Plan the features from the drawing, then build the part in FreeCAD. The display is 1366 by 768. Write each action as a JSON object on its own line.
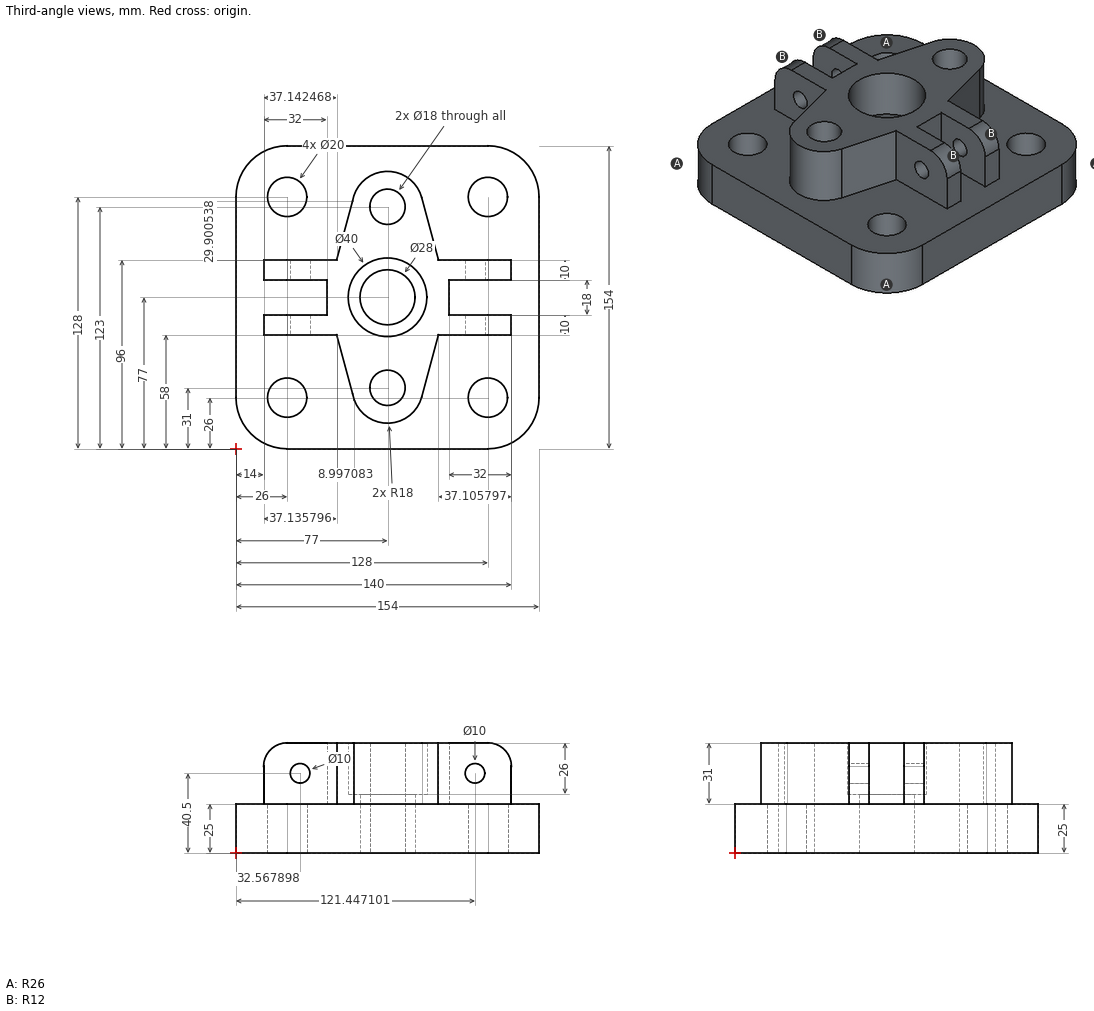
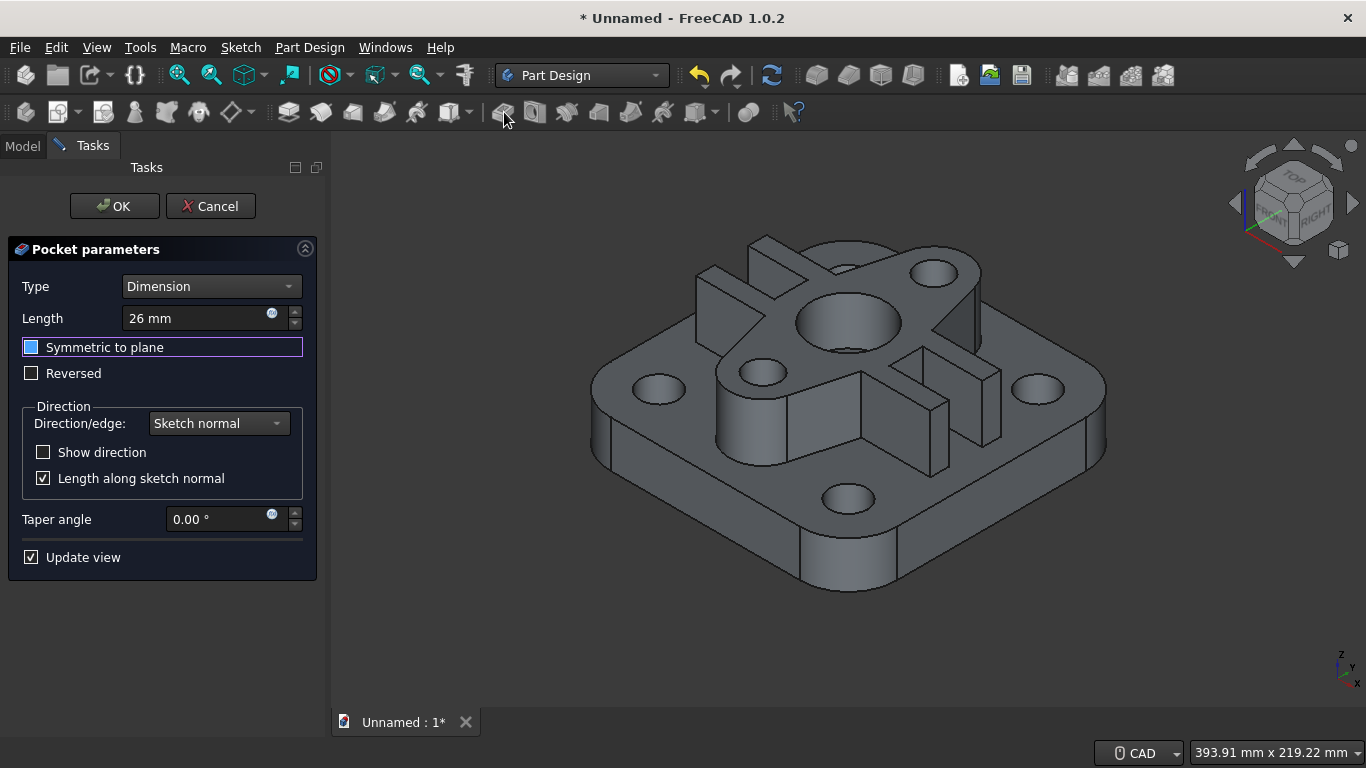
{"action": "left_click", "coordinate": [115, 206]}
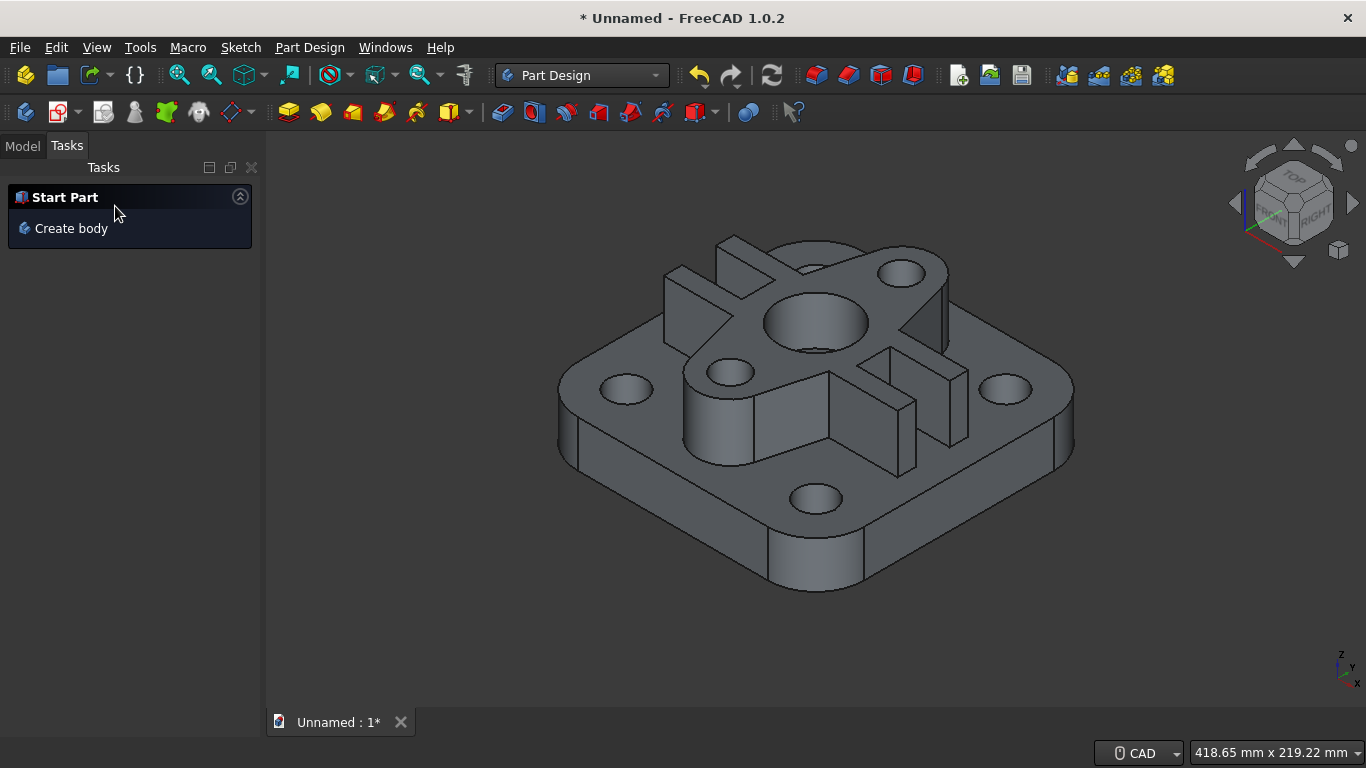
{"action": "left_click", "coordinate": [698, 328]}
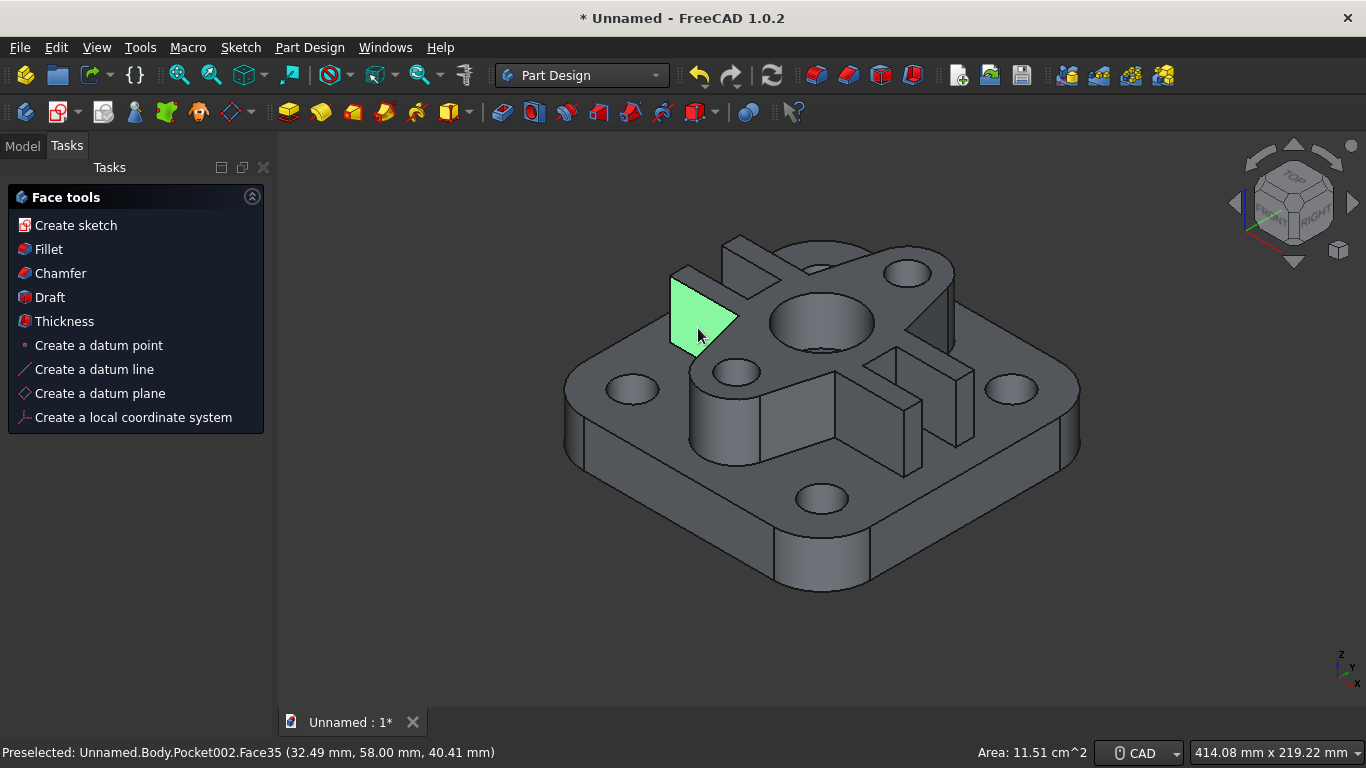
{"action": "left_click", "coordinate": [58, 112]}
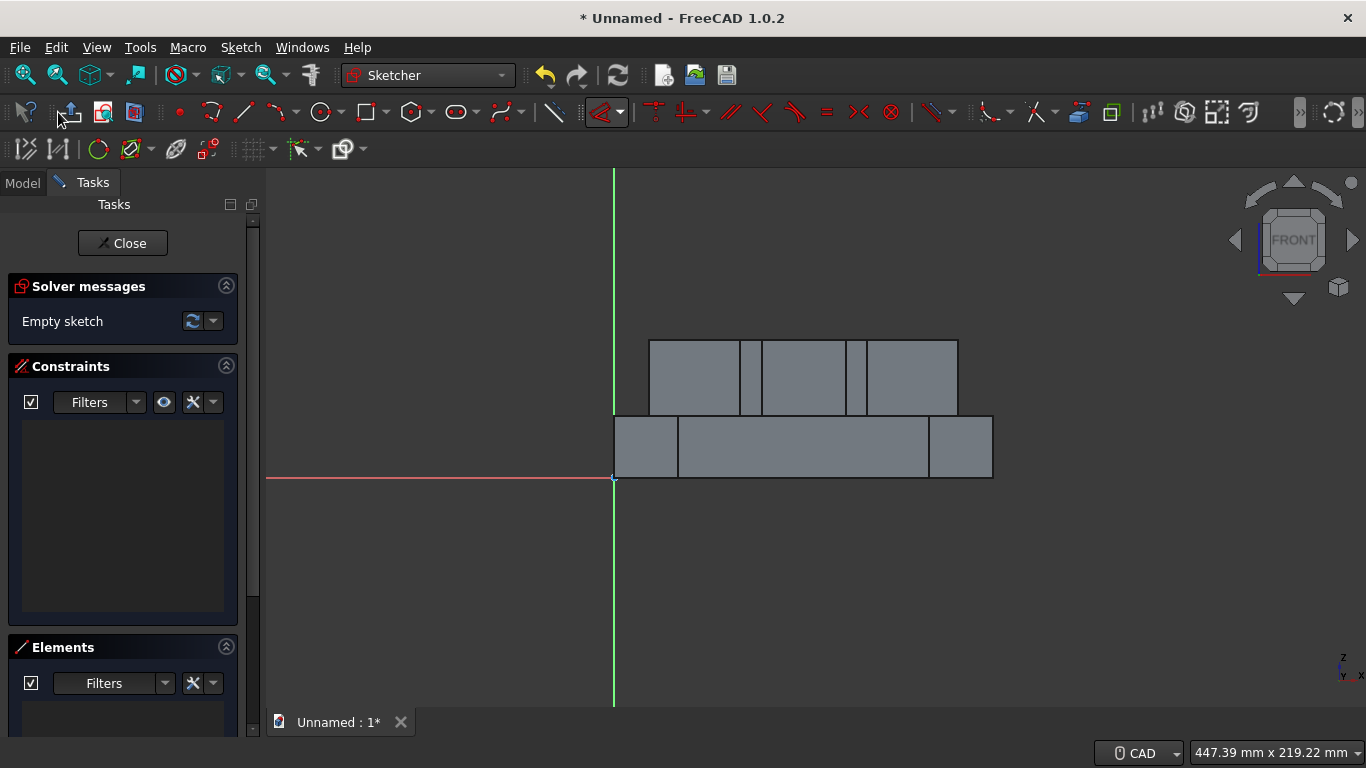
{"action": "scroll", "coordinate": [690, 373], "scroll_direction": "up", "scroll_amount": 13}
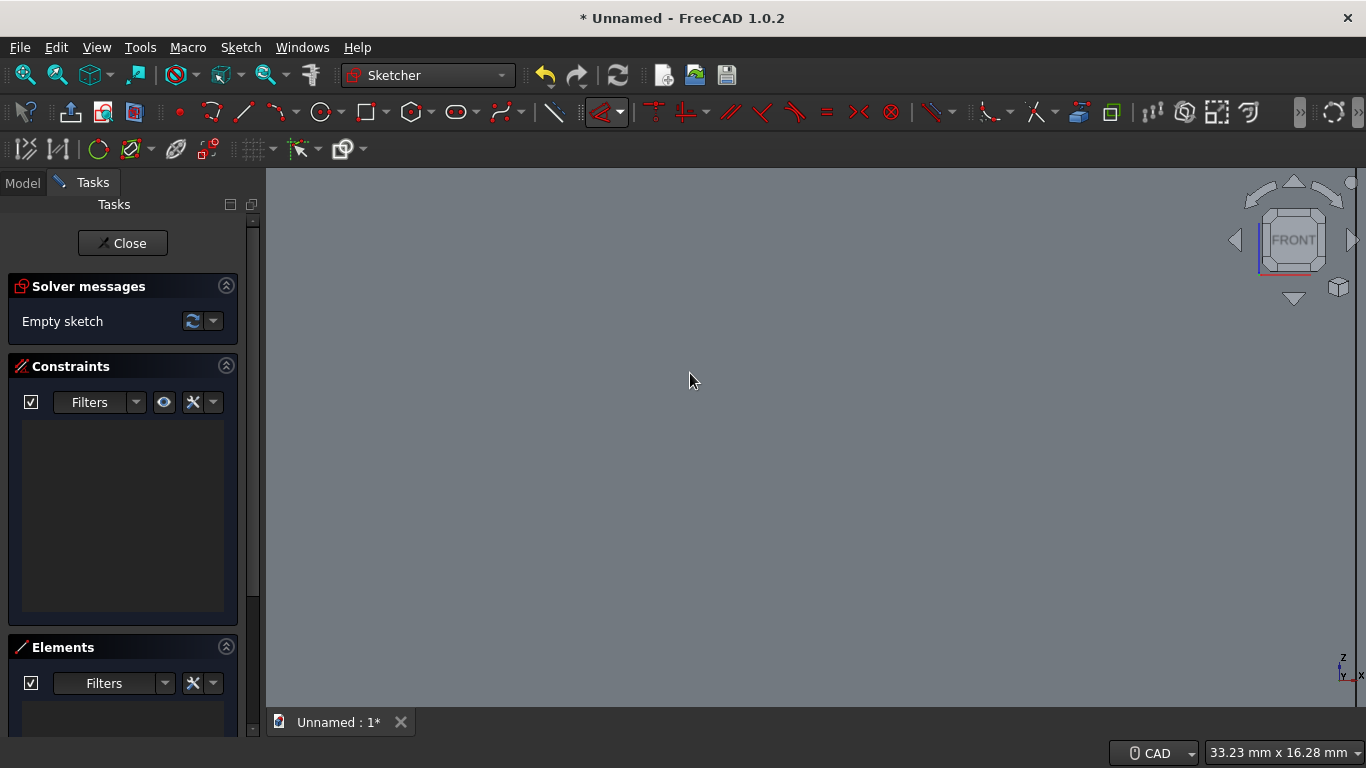
{"action": "left_click", "coordinate": [322, 112]}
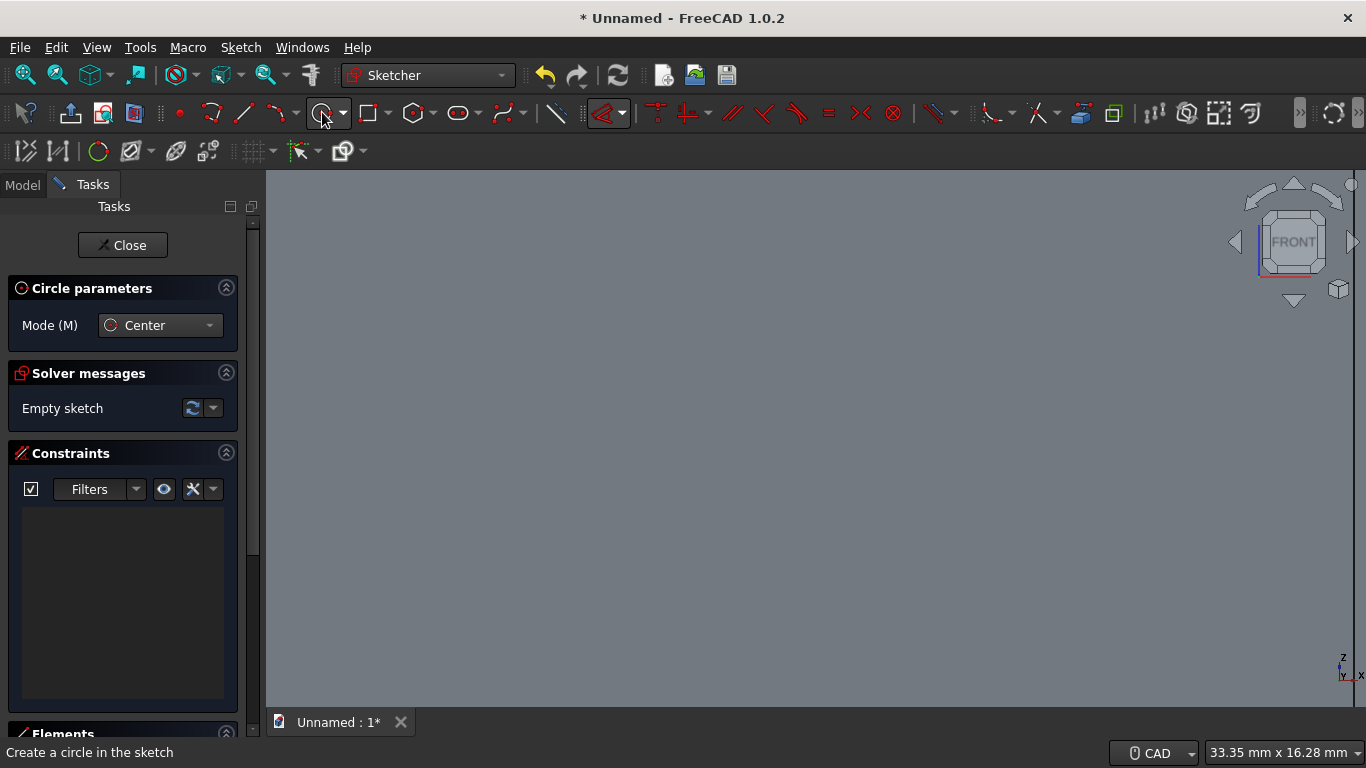
{"action": "left_click", "coordinate": [742, 437]}
{"action": "left_click", "coordinate": [858, 321]}
{"action": "key", "text": "Escape"}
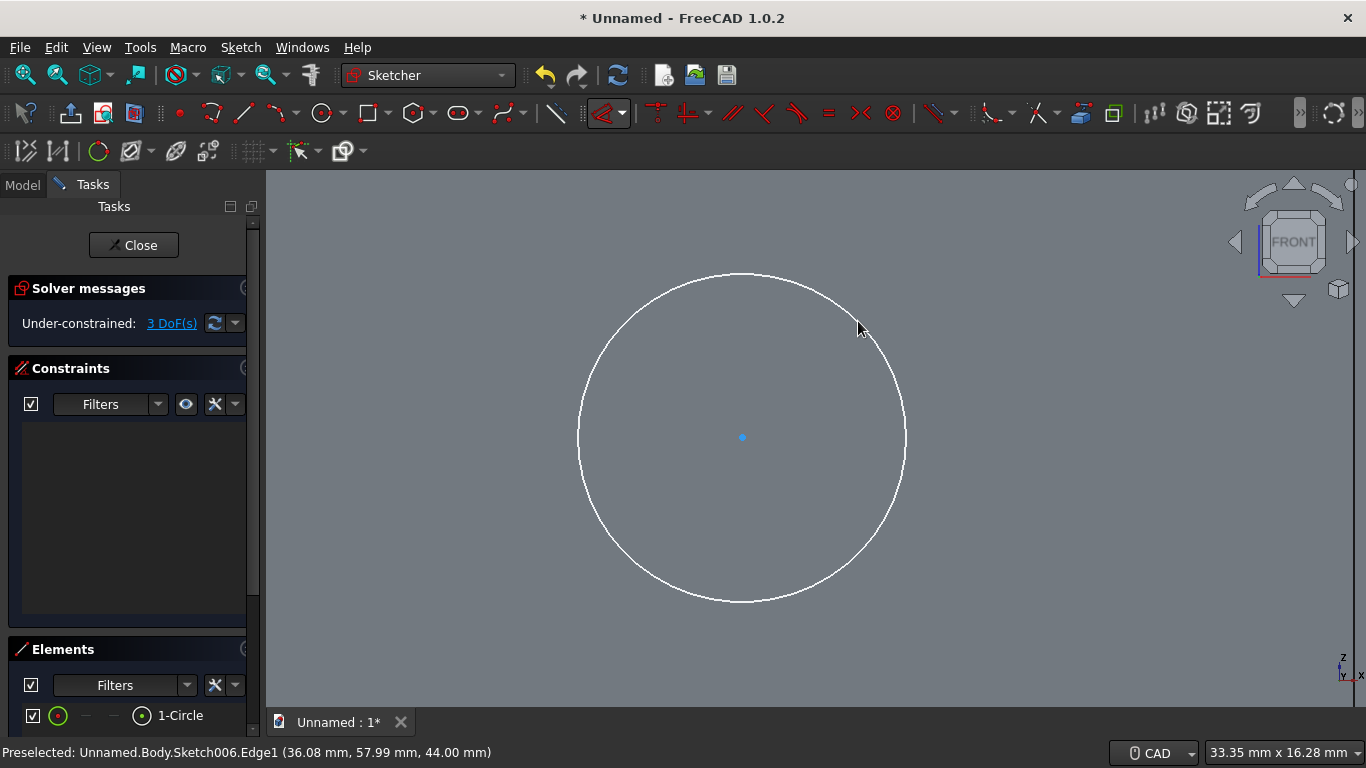
{"action": "left_click", "coordinate": [858, 322]}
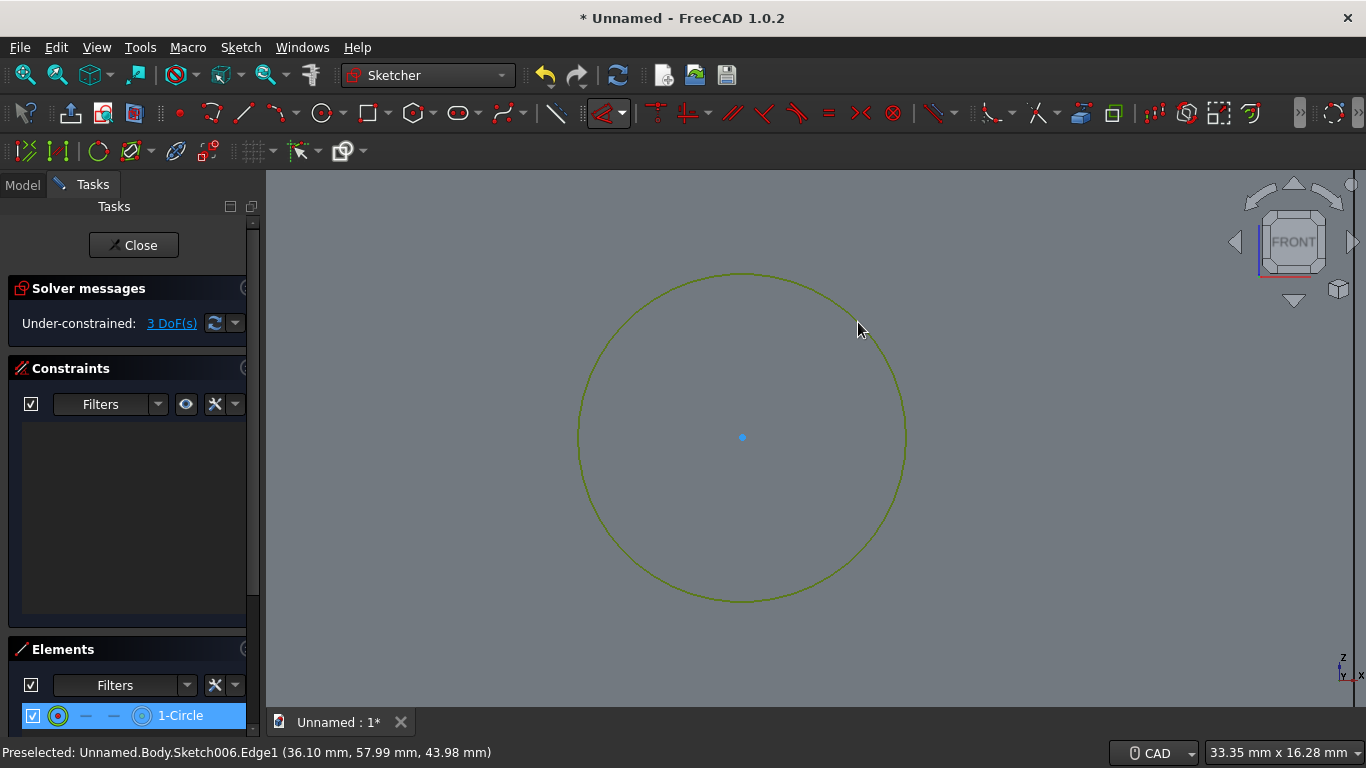
{"action": "left_click", "coordinate": [624, 114]}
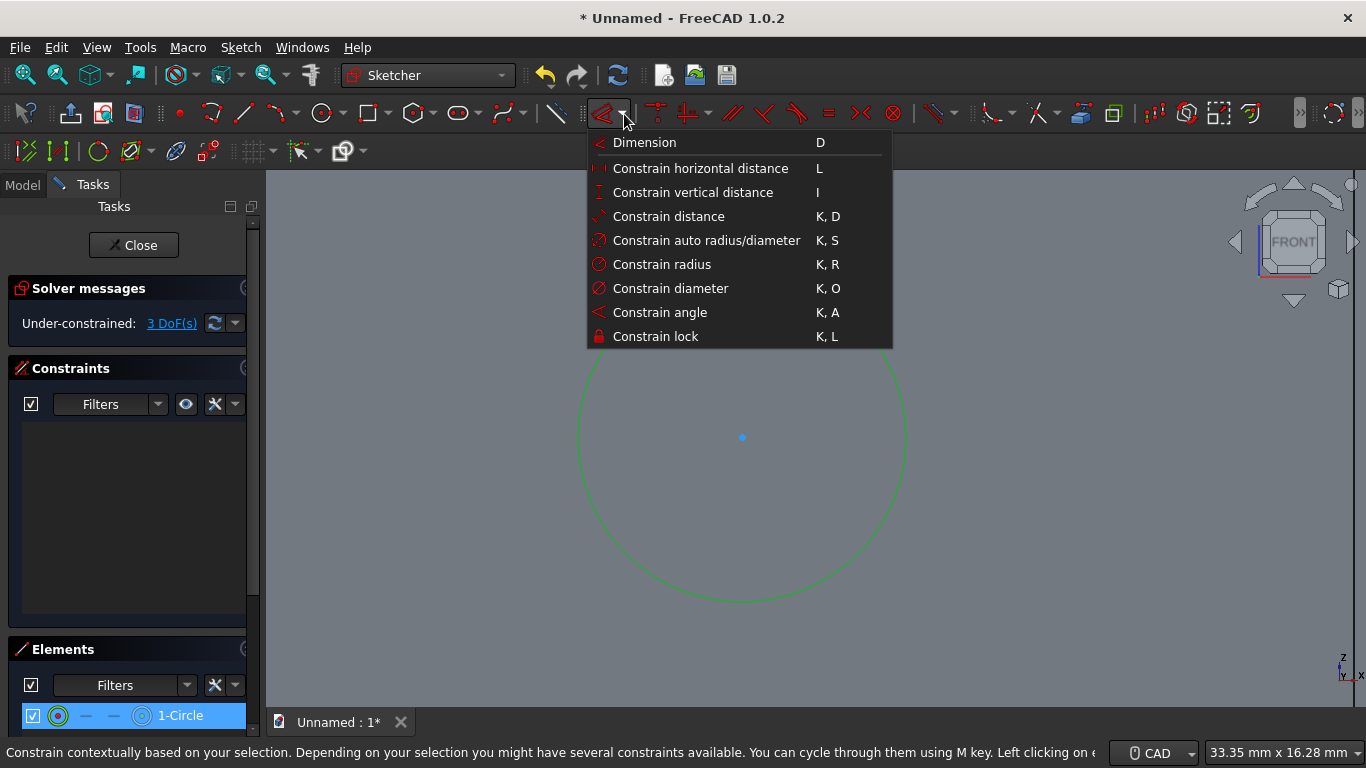
{"action": "left_click", "coordinate": [740, 288]}